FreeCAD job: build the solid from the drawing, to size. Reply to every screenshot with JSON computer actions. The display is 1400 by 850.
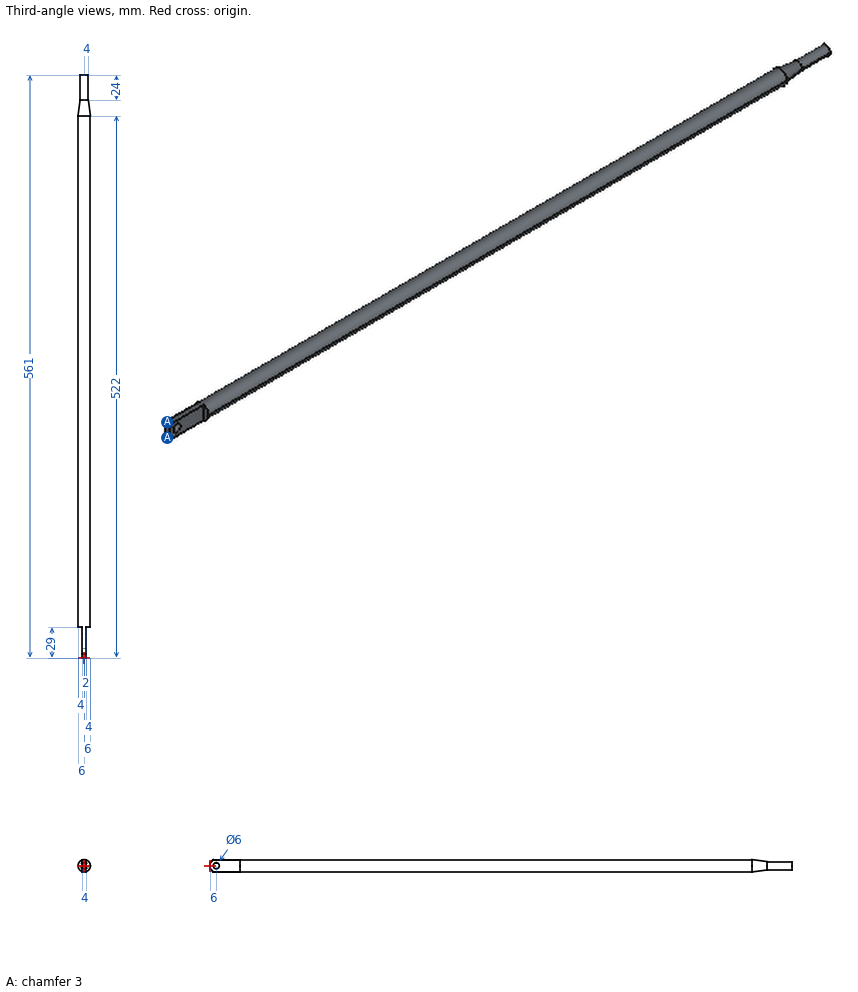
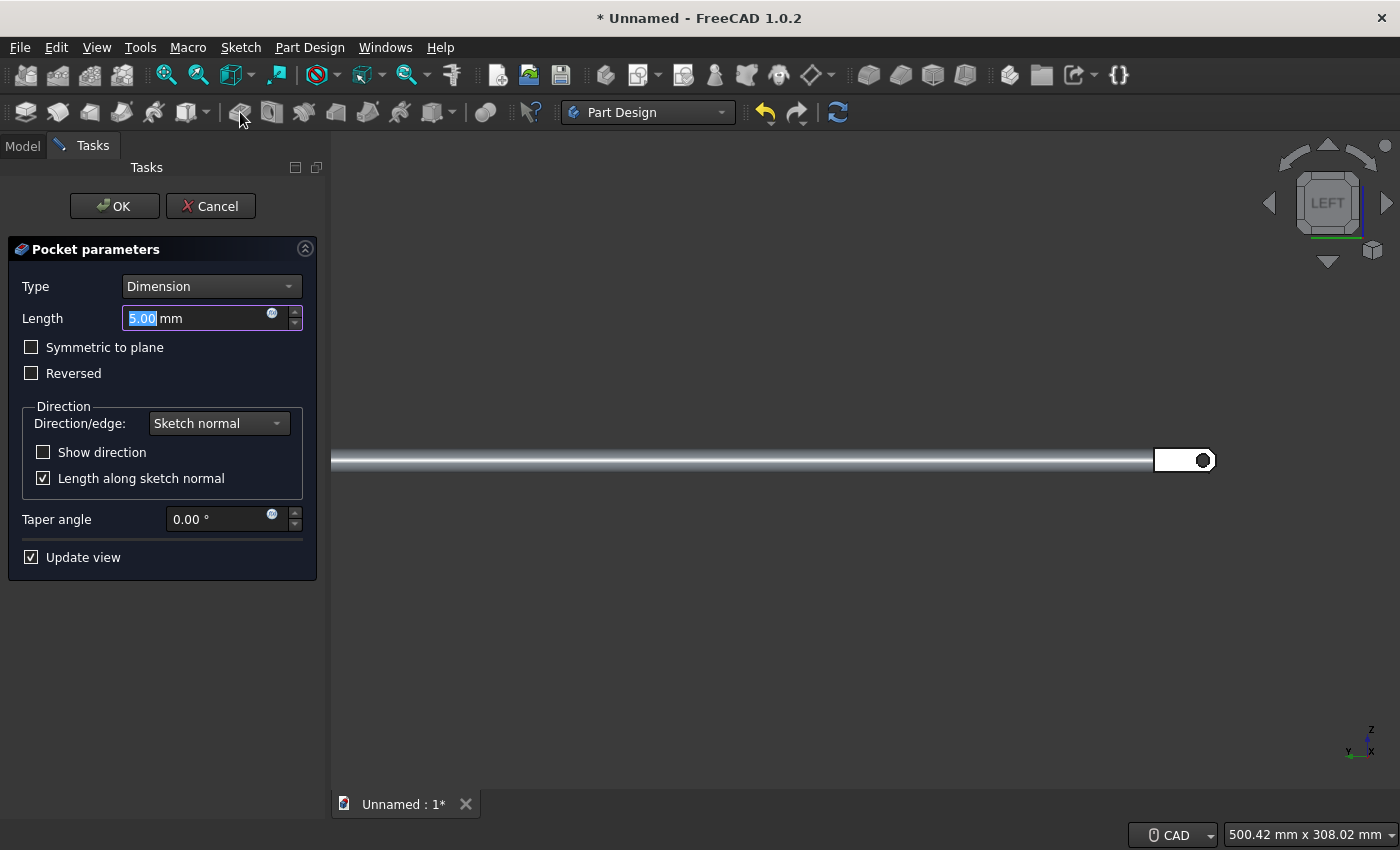
{"action": "type", "text": "4"}
{"action": "key", "text": "Tab"}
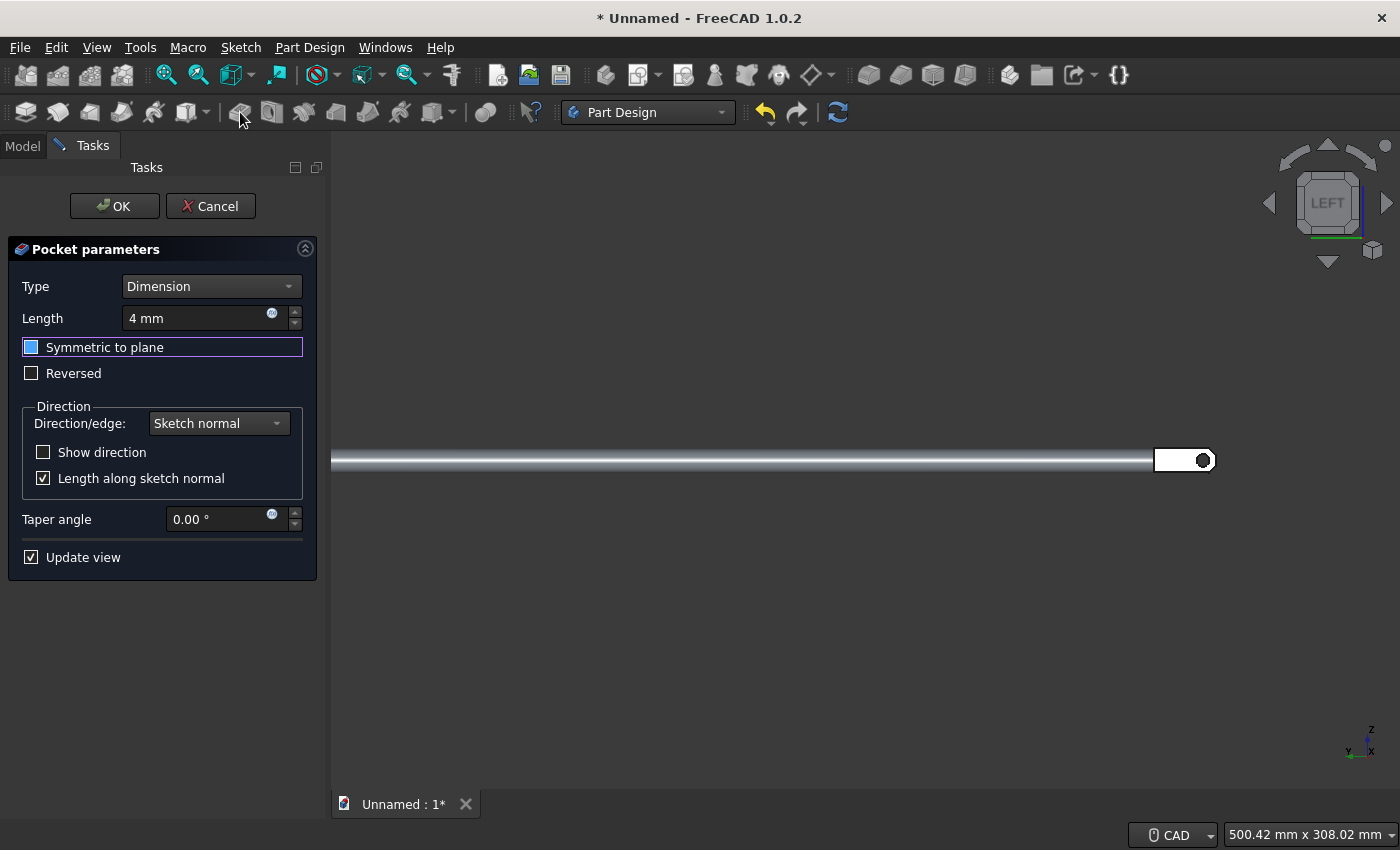
{"action": "left_click", "coordinate": [115, 206]}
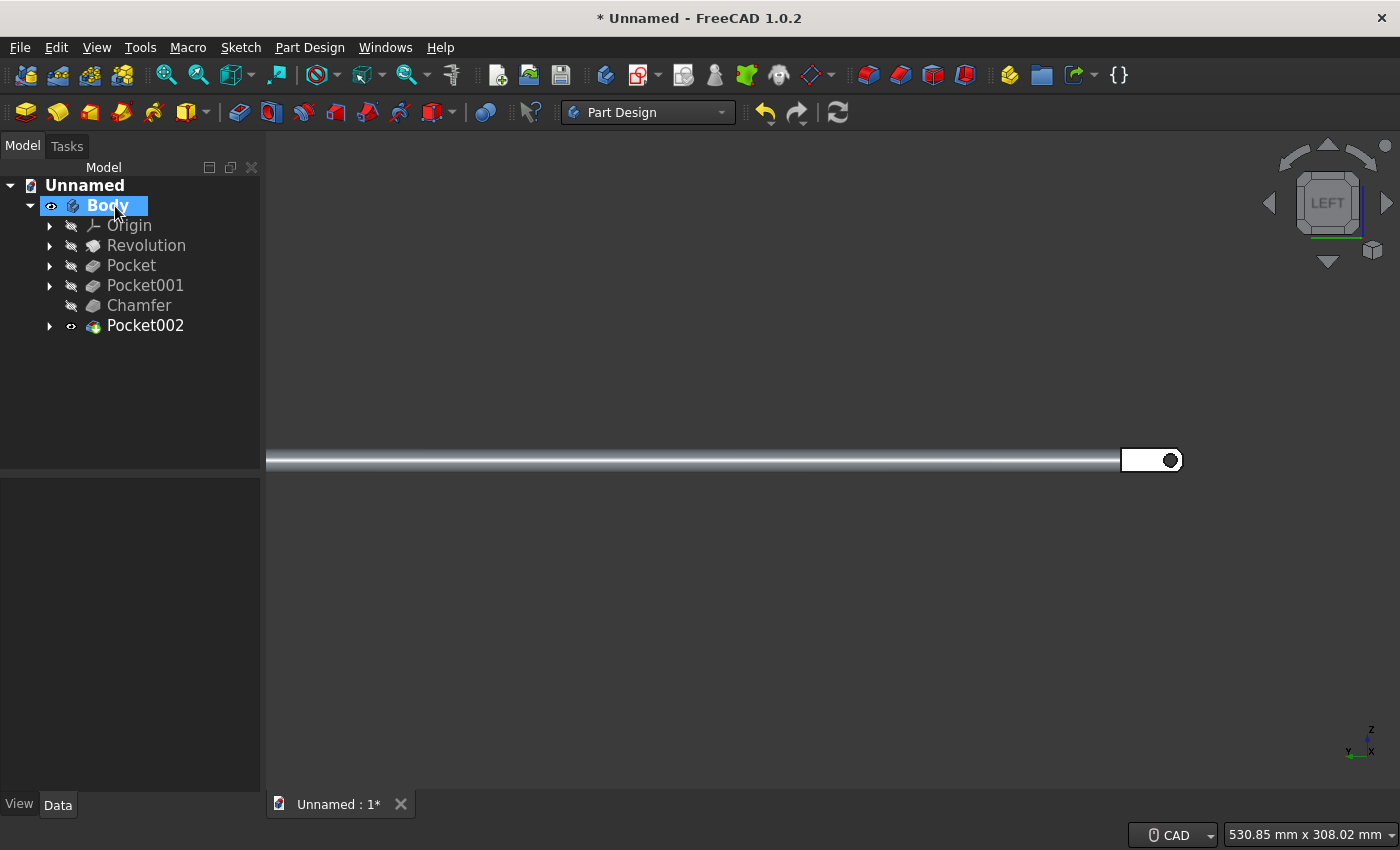
{"action": "key", "text": "0"}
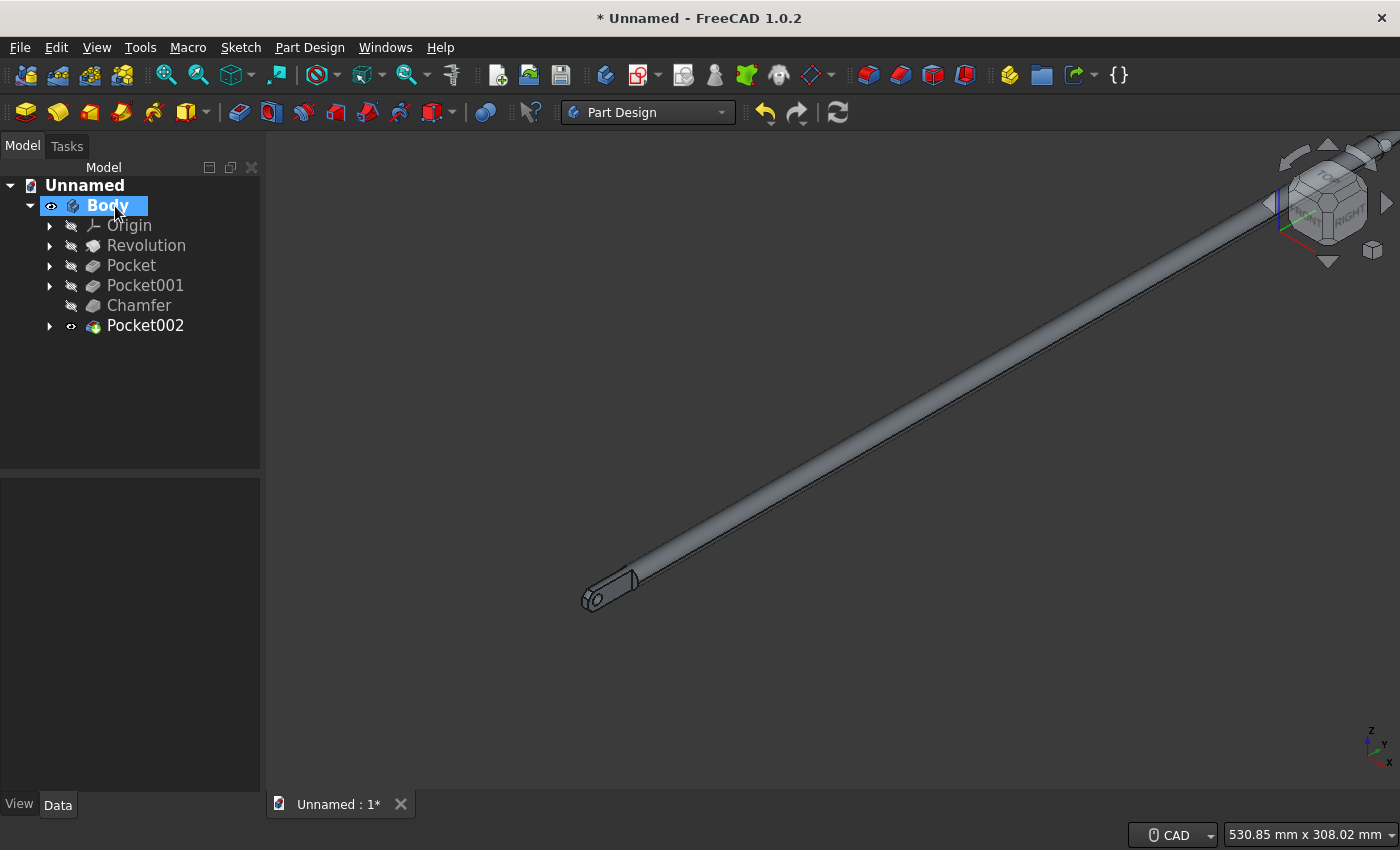
{"action": "left_click", "coordinate": [168, 76]}